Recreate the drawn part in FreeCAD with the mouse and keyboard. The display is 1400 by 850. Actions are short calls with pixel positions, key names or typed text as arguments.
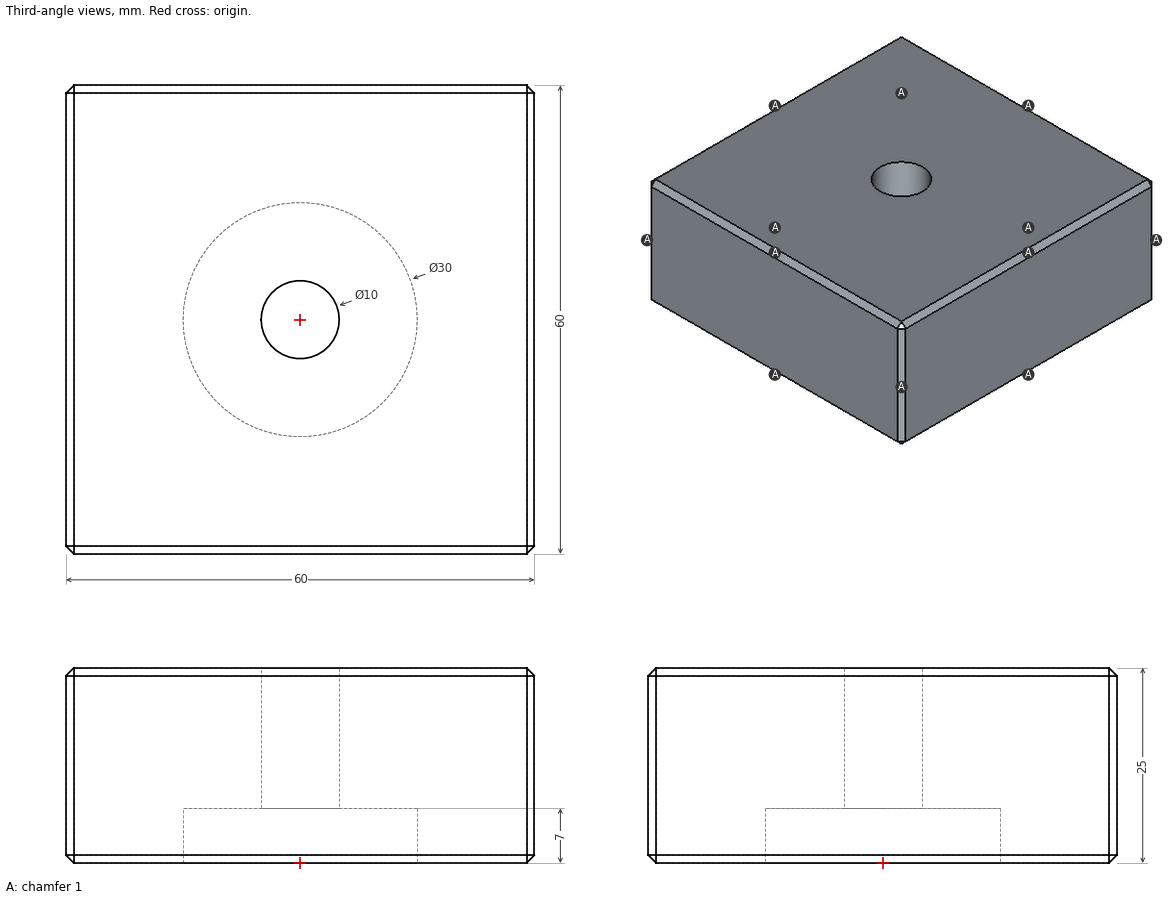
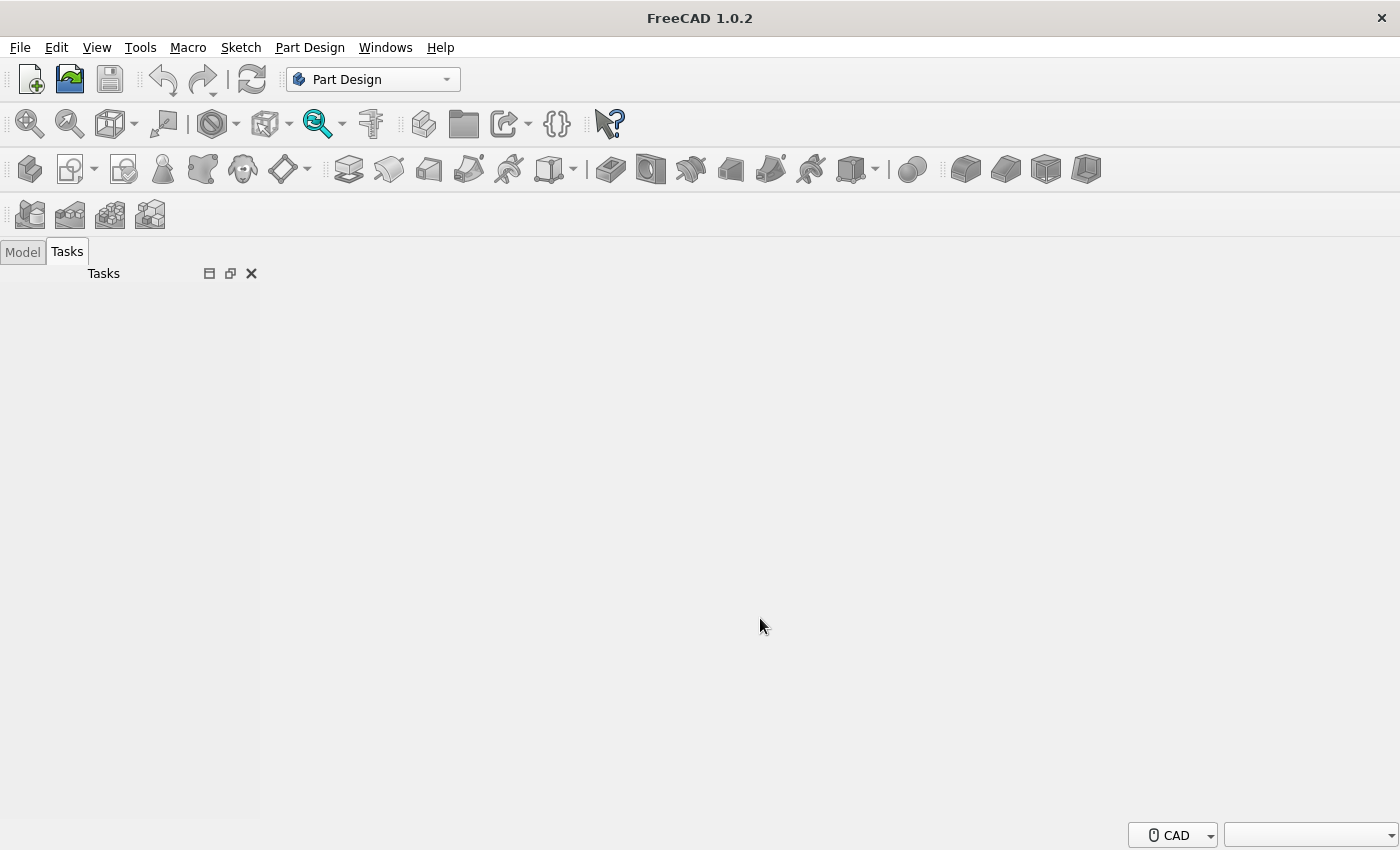
key(ctrl+n)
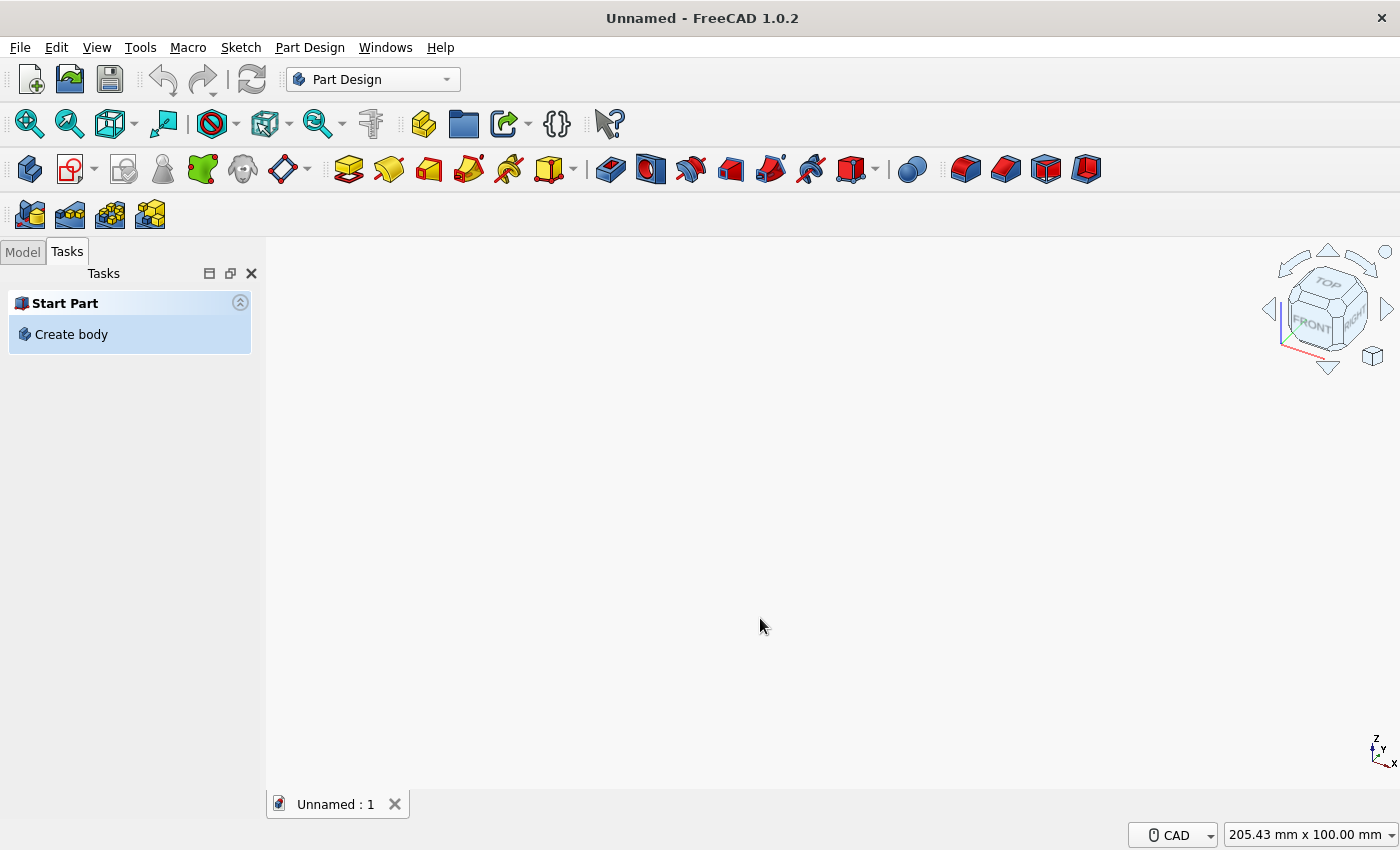
click(70, 170)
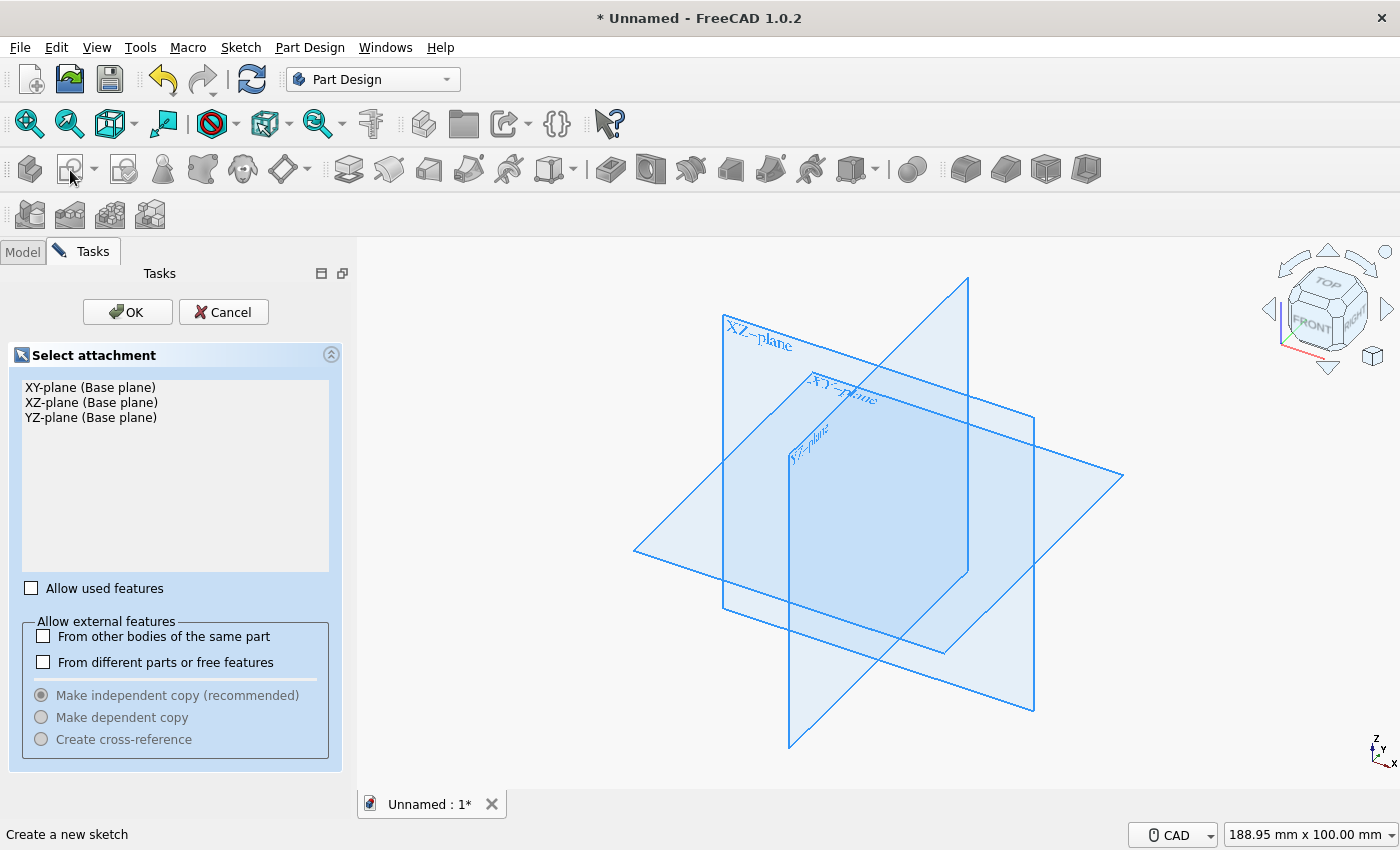
click(82, 388)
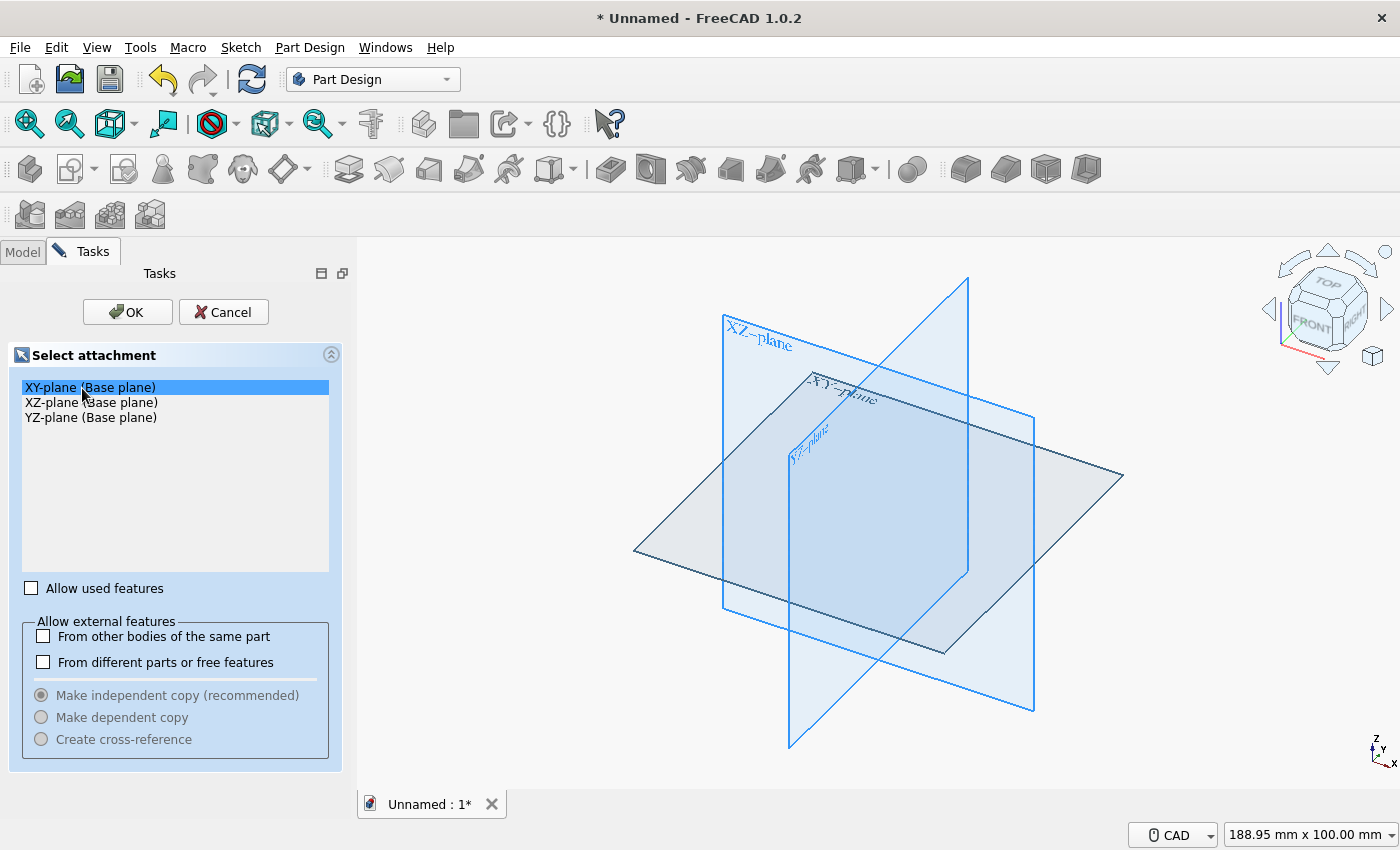
click(128, 312)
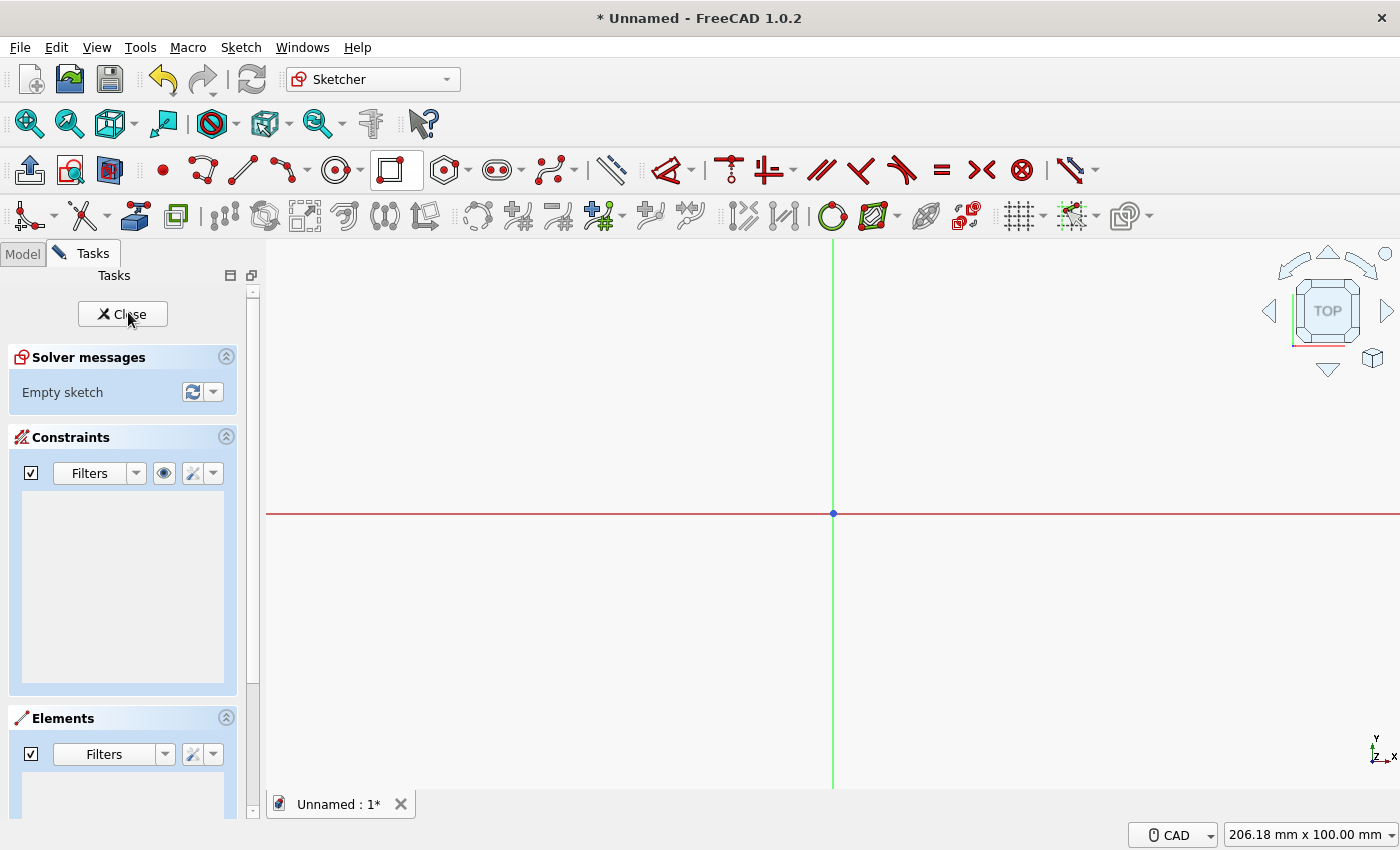
click(418, 170)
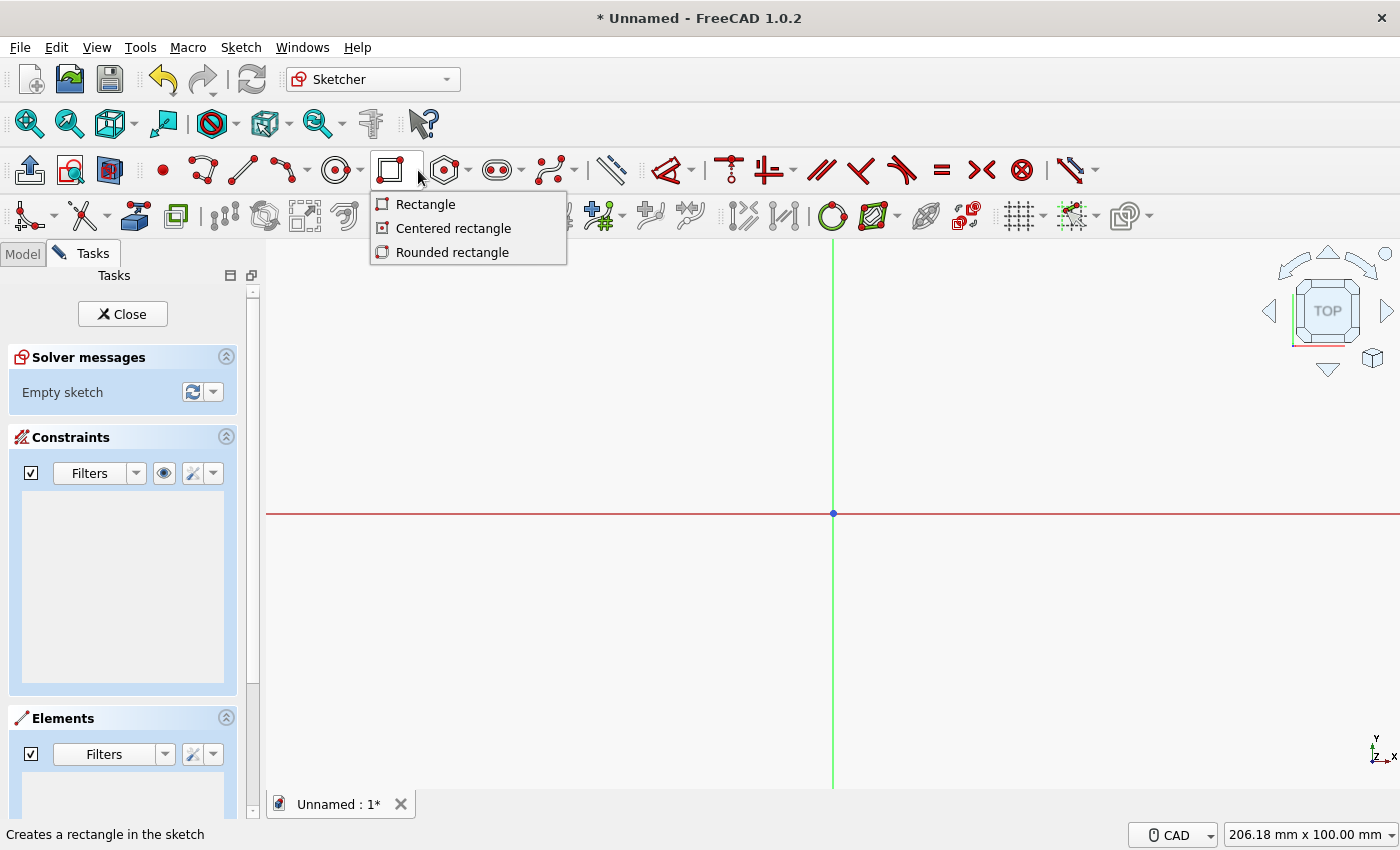
click(468, 228)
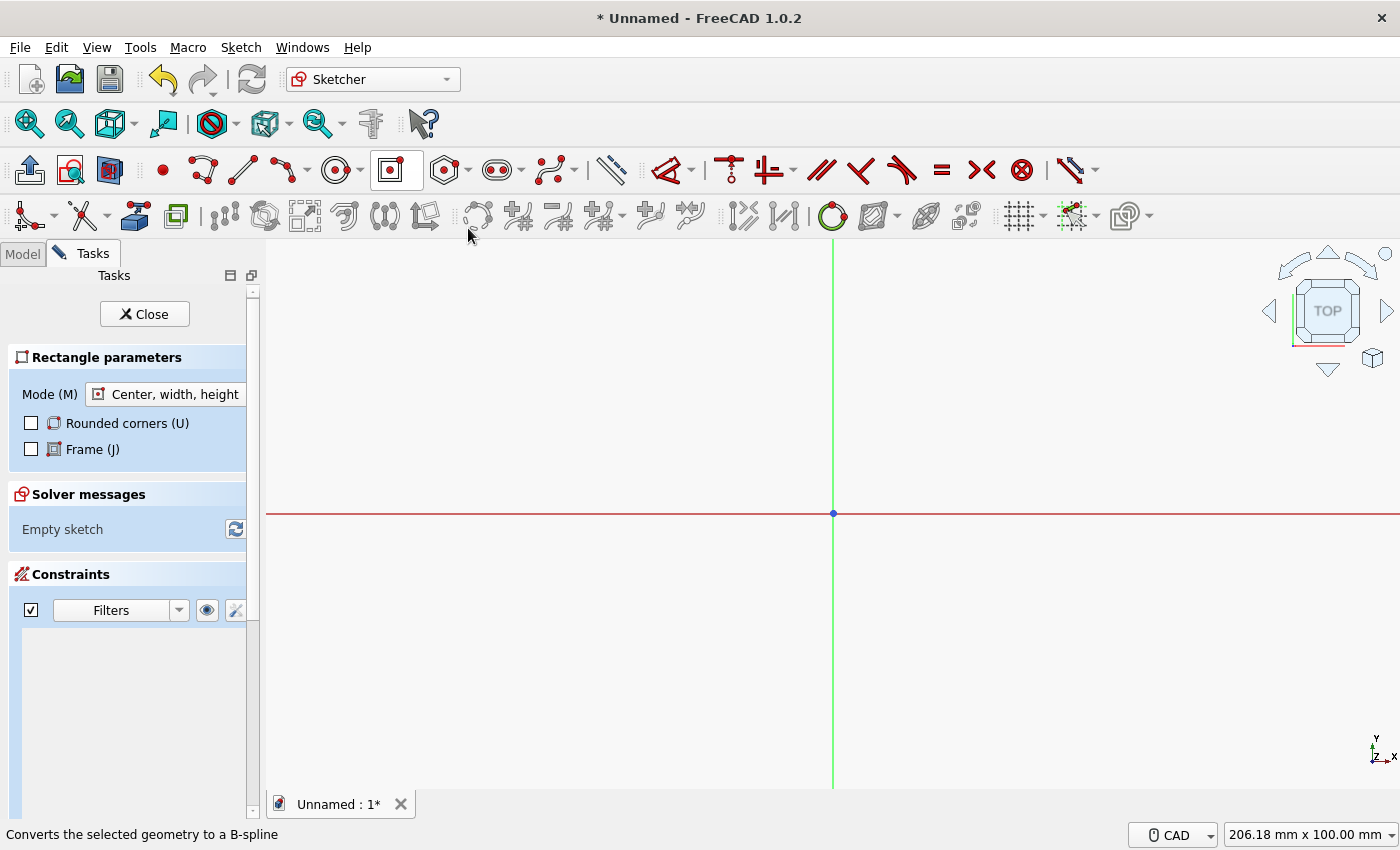
click(833, 514)
move(998, 349)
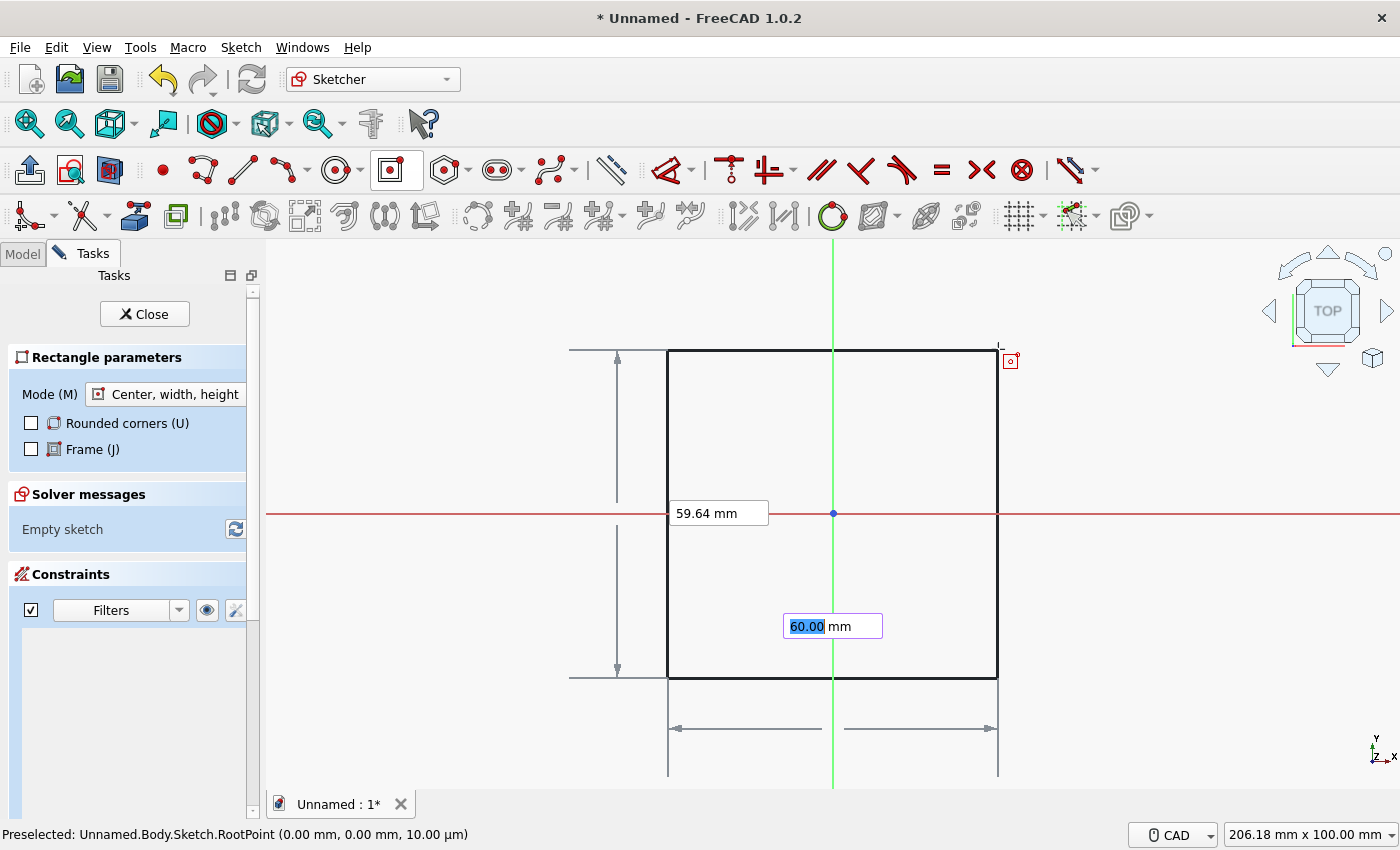
text(60)
key(Tab)
text(60)
key(Return)
key(Escape)